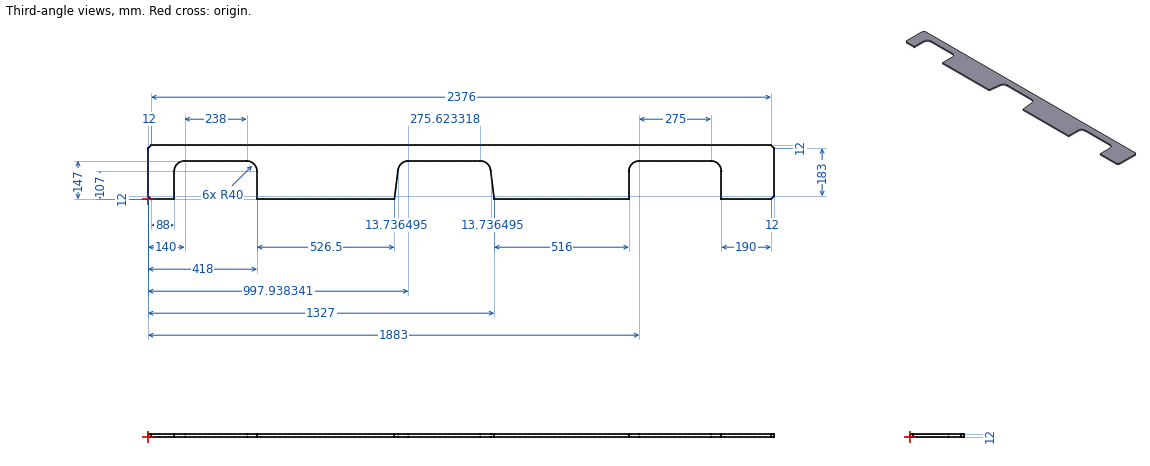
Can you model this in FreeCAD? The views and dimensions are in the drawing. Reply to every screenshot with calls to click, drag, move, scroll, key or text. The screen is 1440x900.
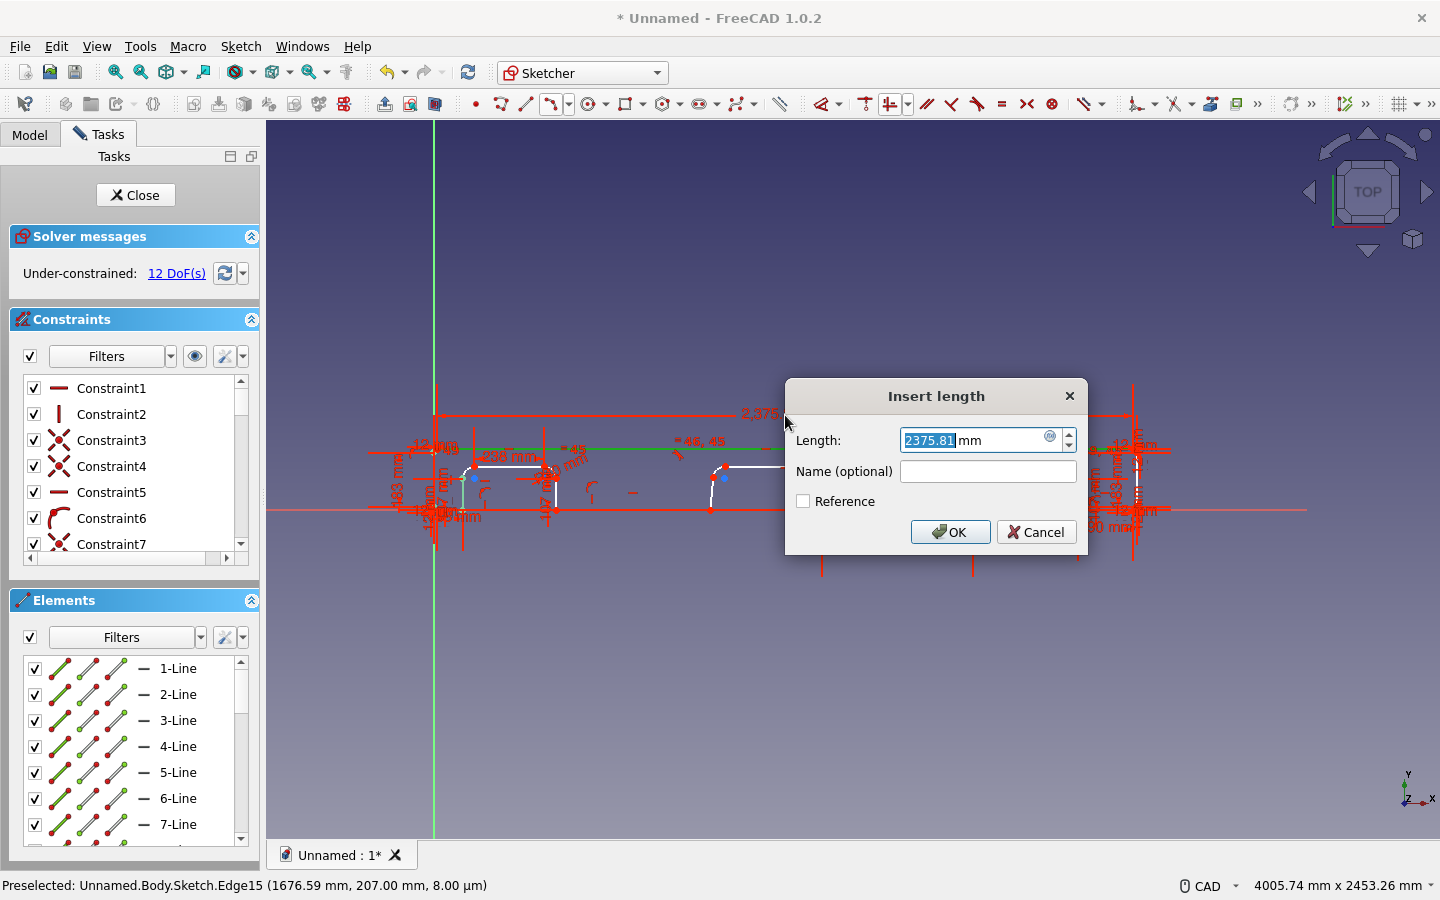
text(2376)
key(Return)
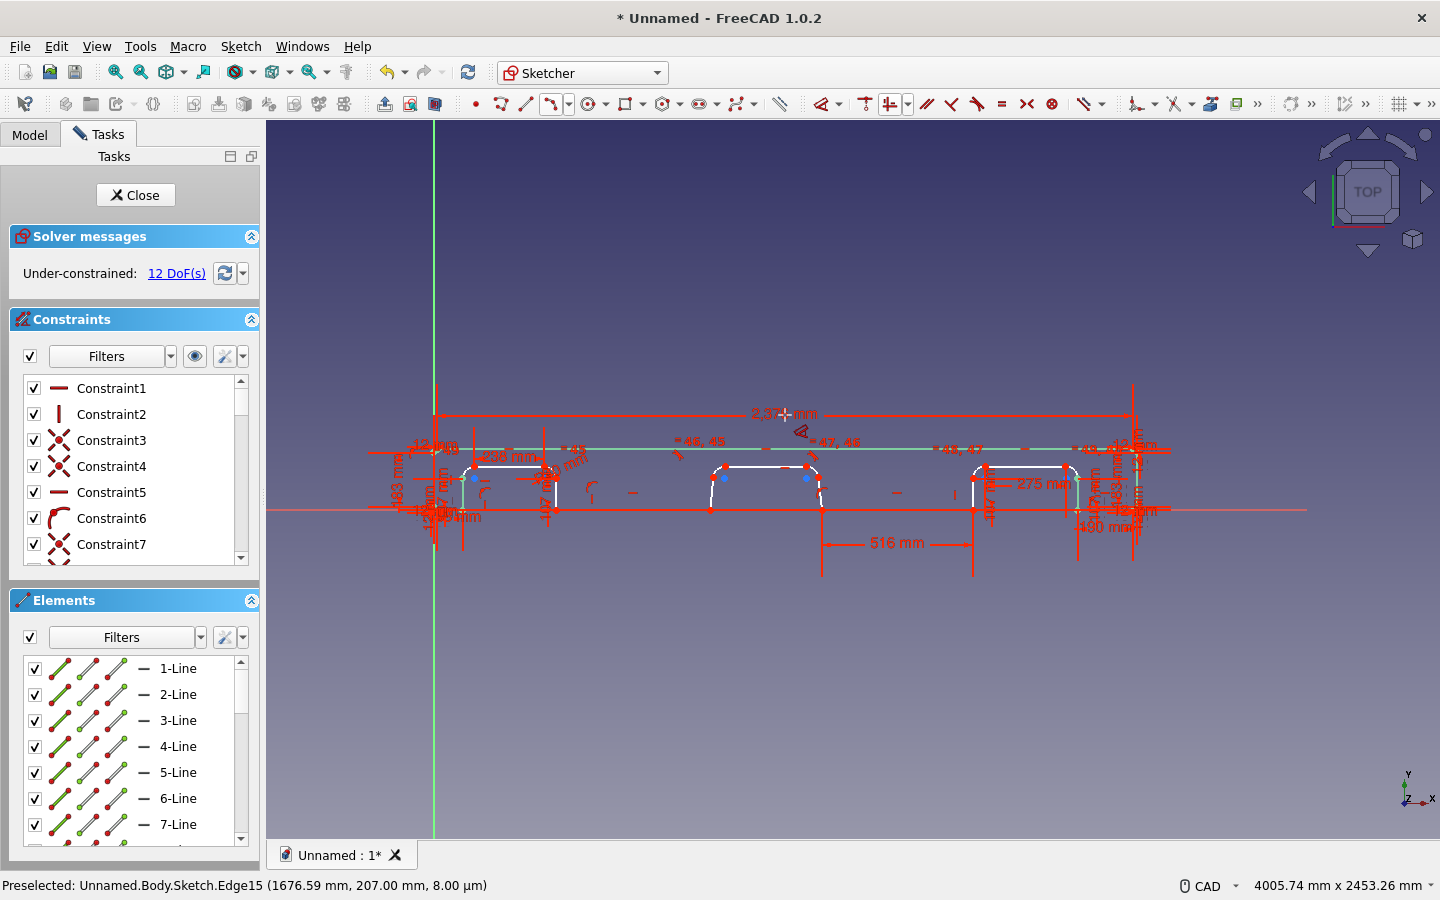
click(474, 467)
click(454, 544)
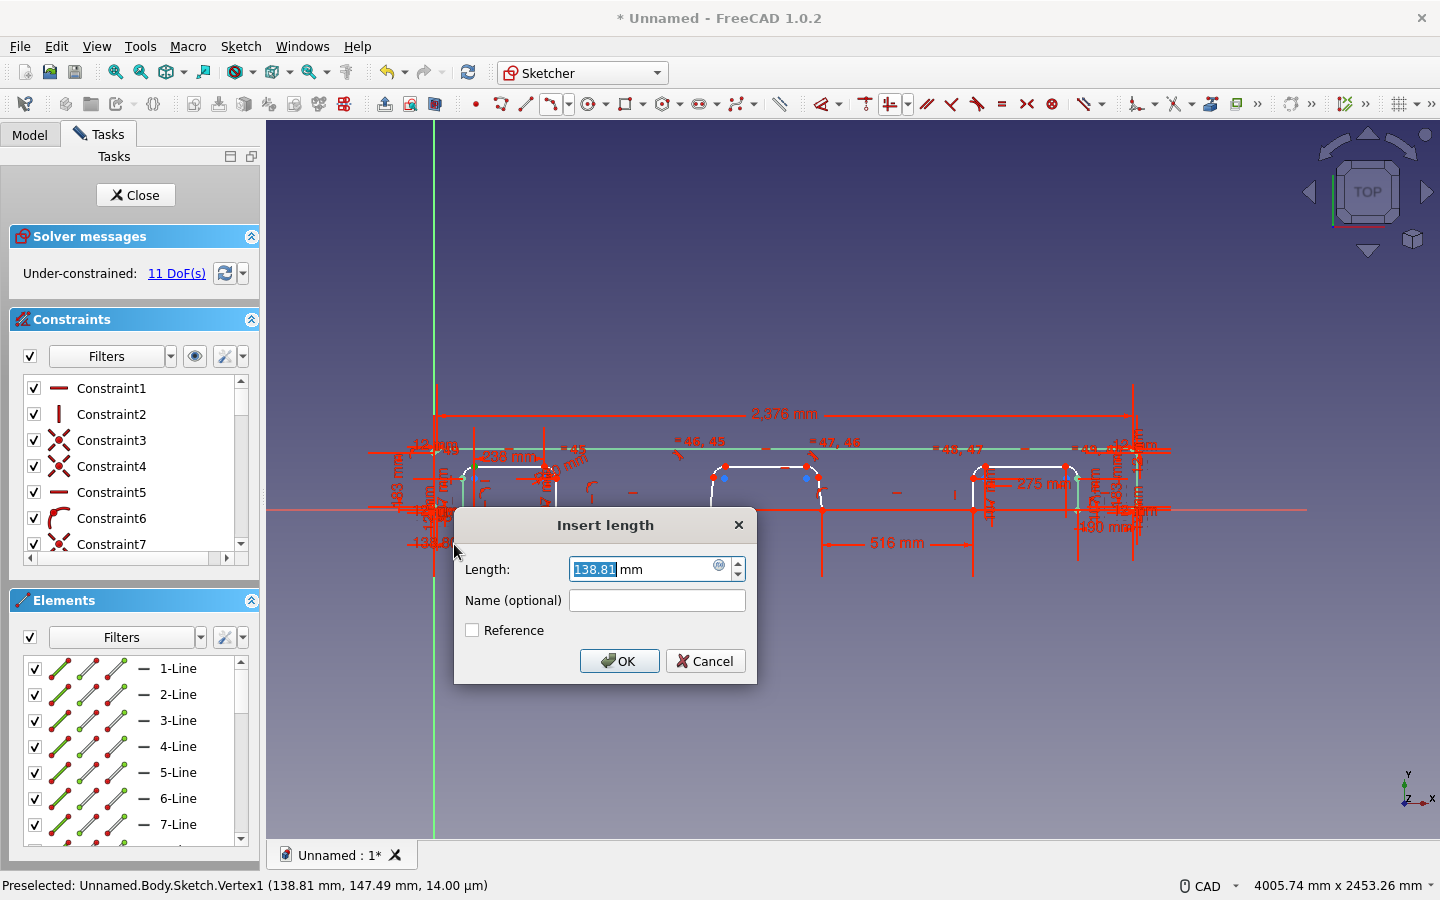
text(140)
key(Return)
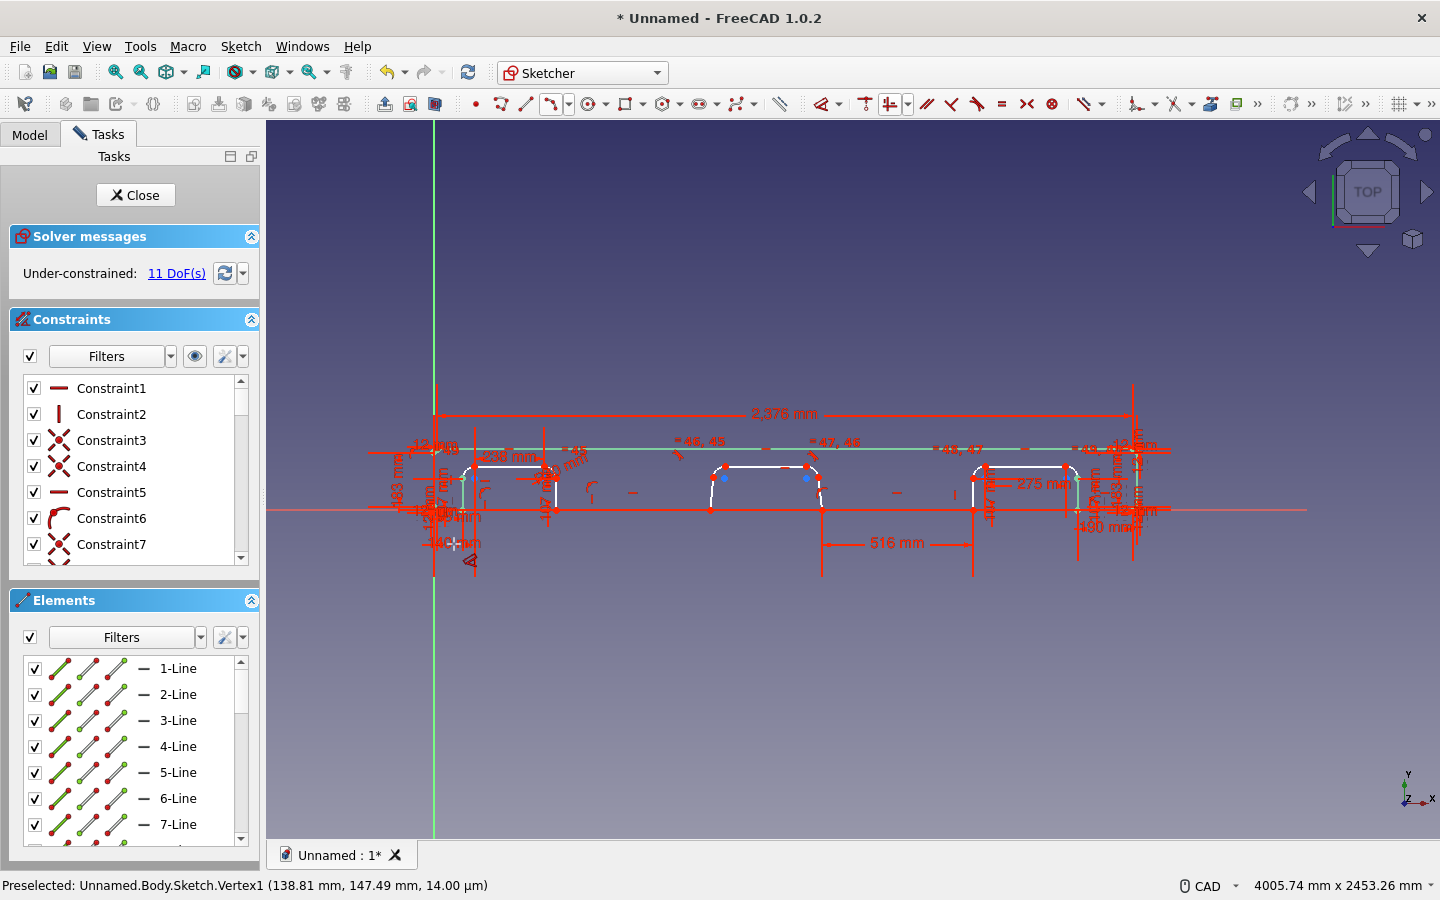
click(475, 467)
click(328, 488)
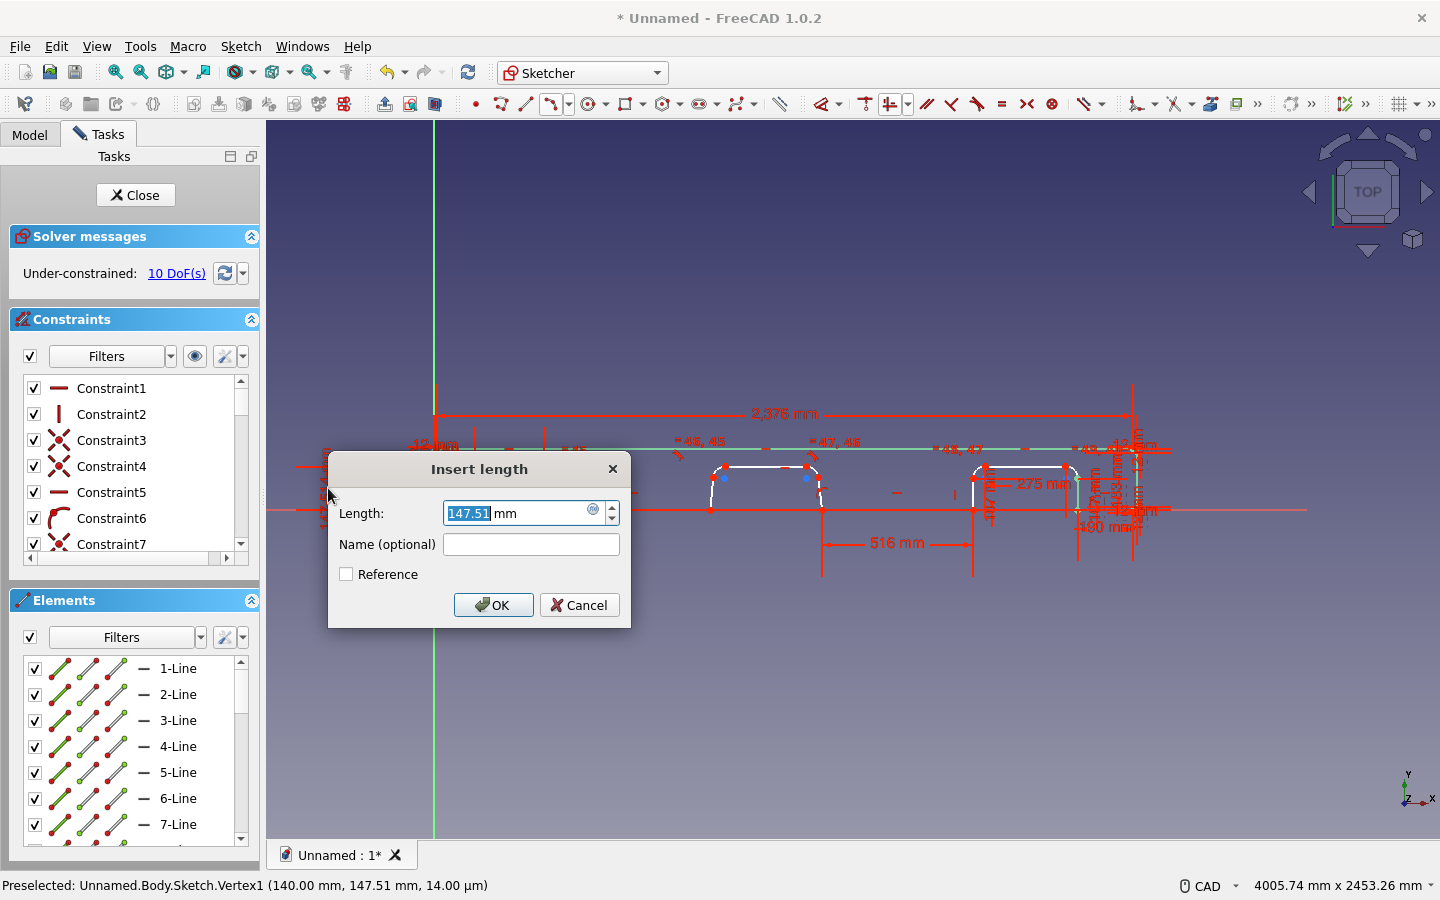
text(147)
key(Return)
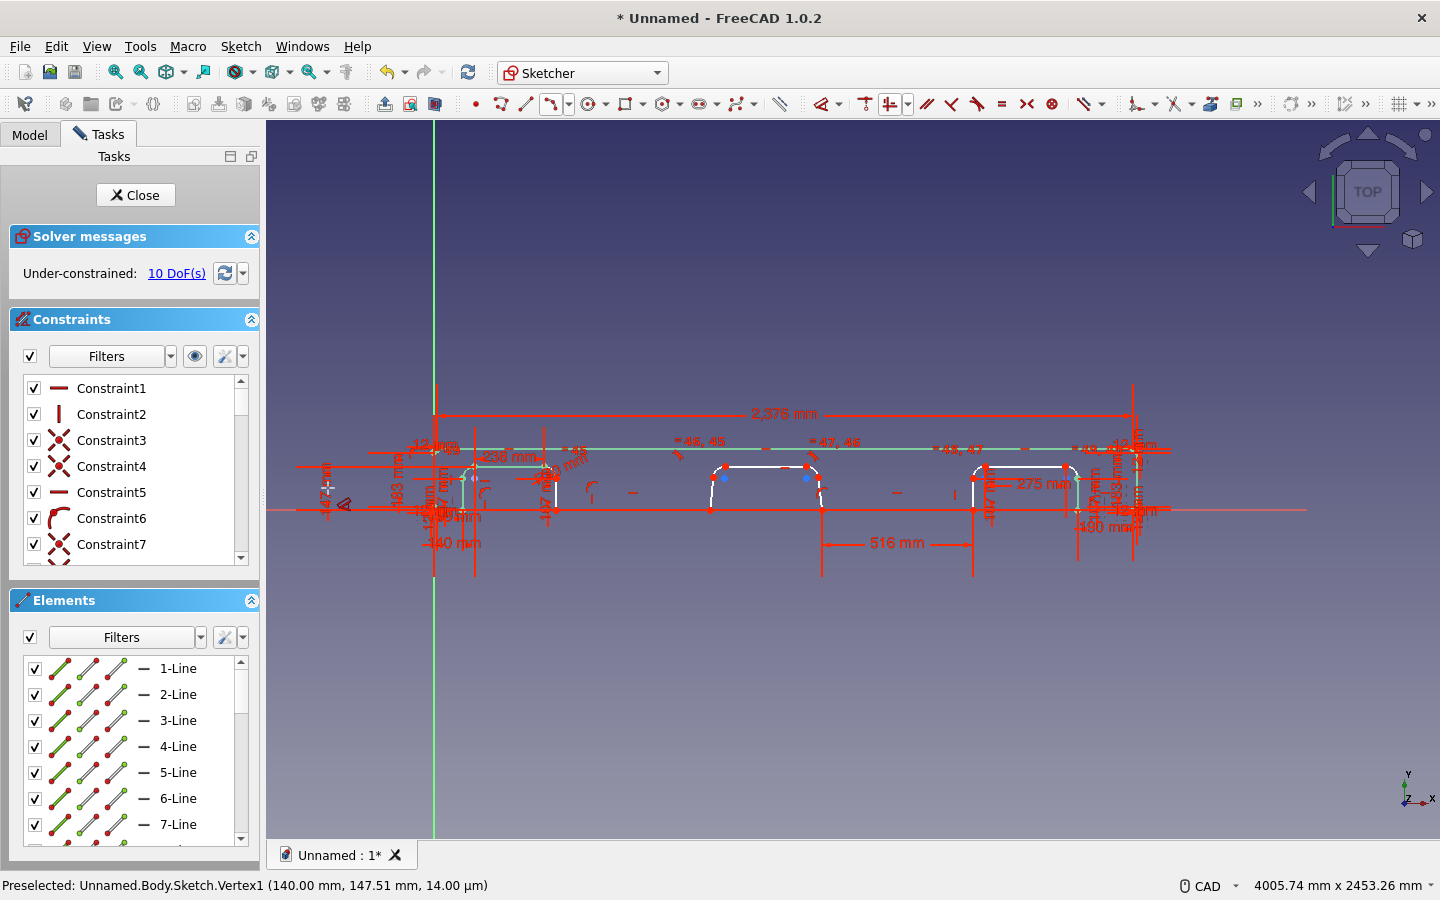
click(556, 479)
click(538, 544)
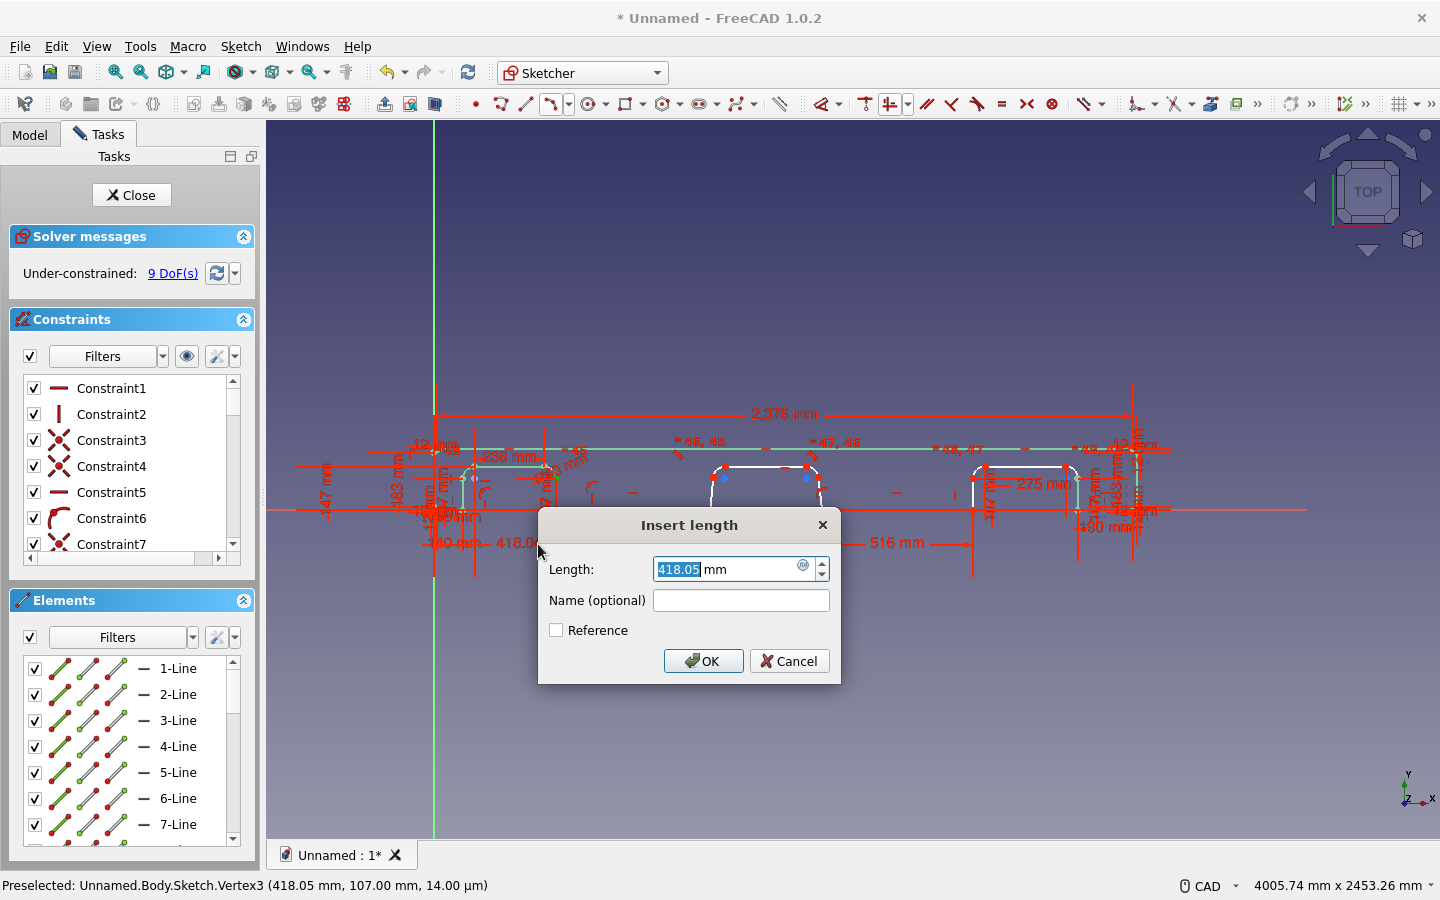
text(418)
key(Return)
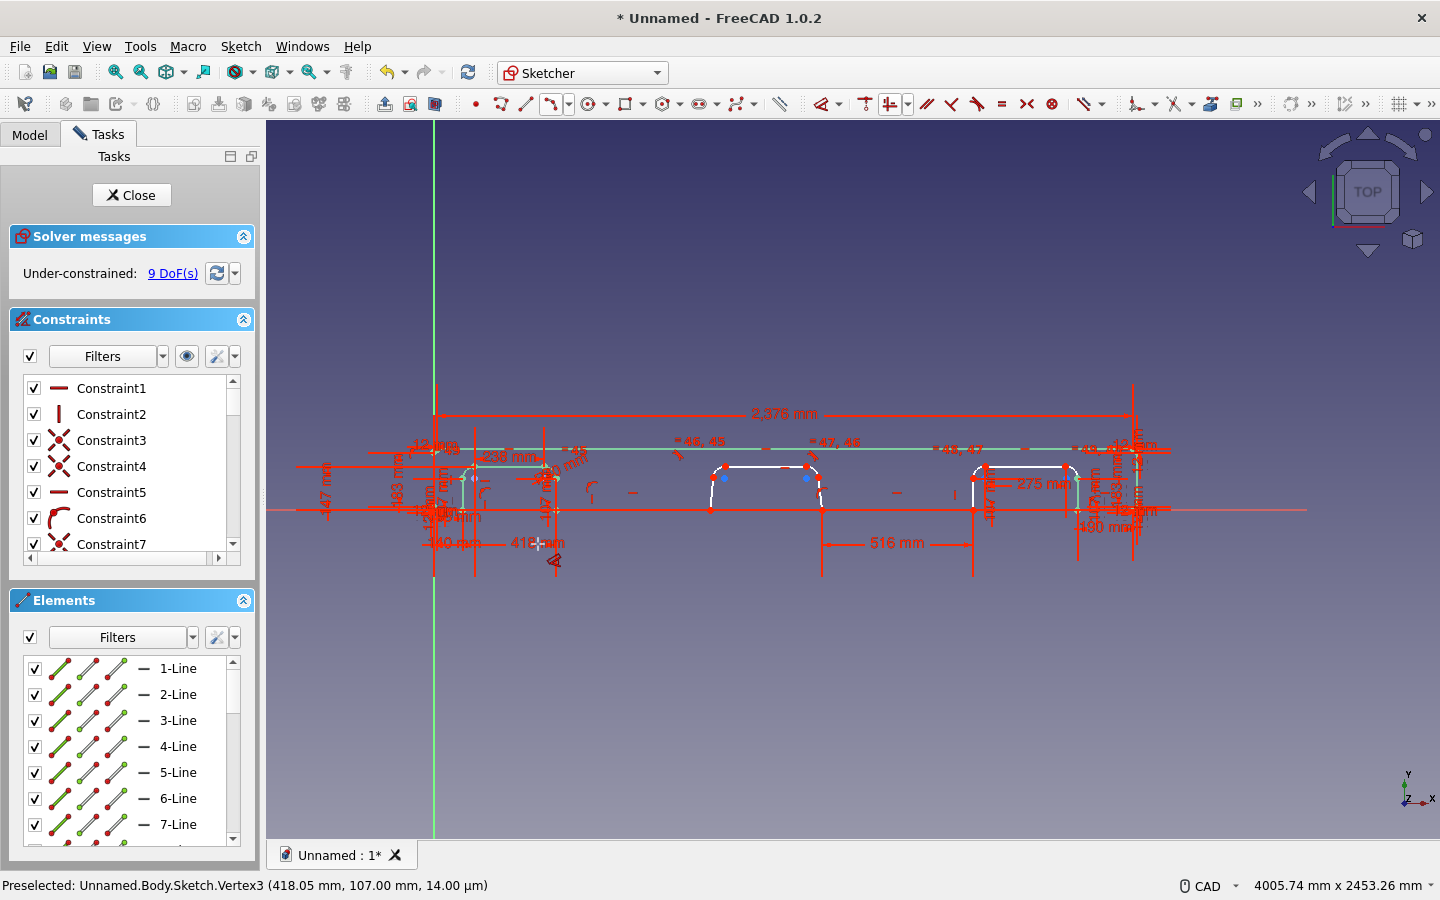
click(726, 467)
click(760, 488)